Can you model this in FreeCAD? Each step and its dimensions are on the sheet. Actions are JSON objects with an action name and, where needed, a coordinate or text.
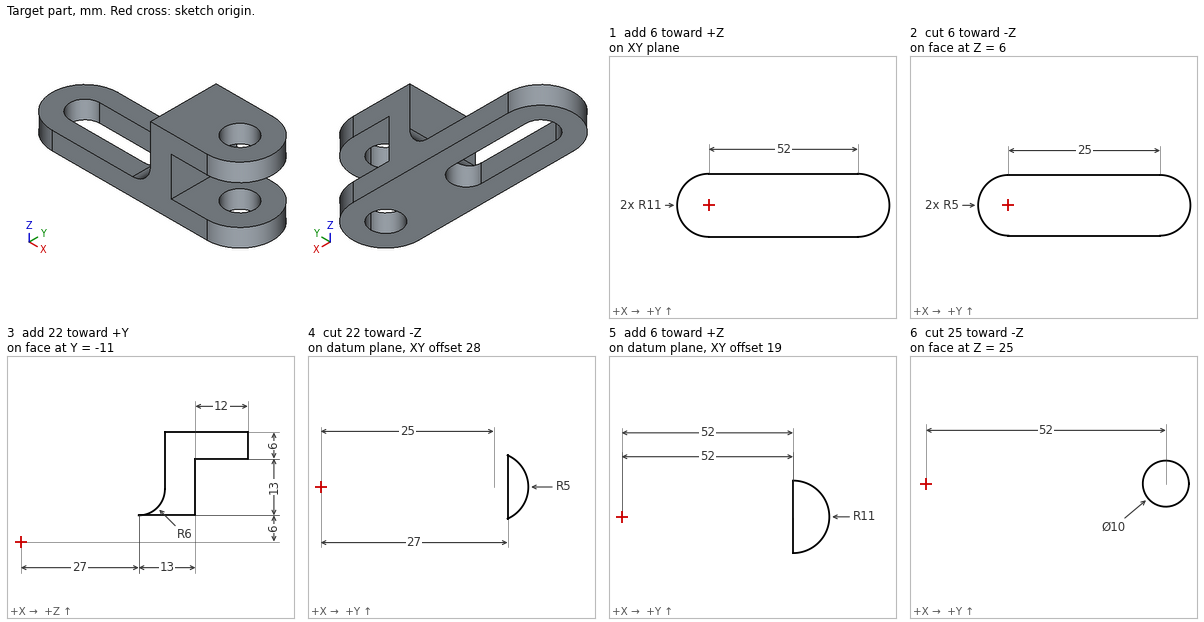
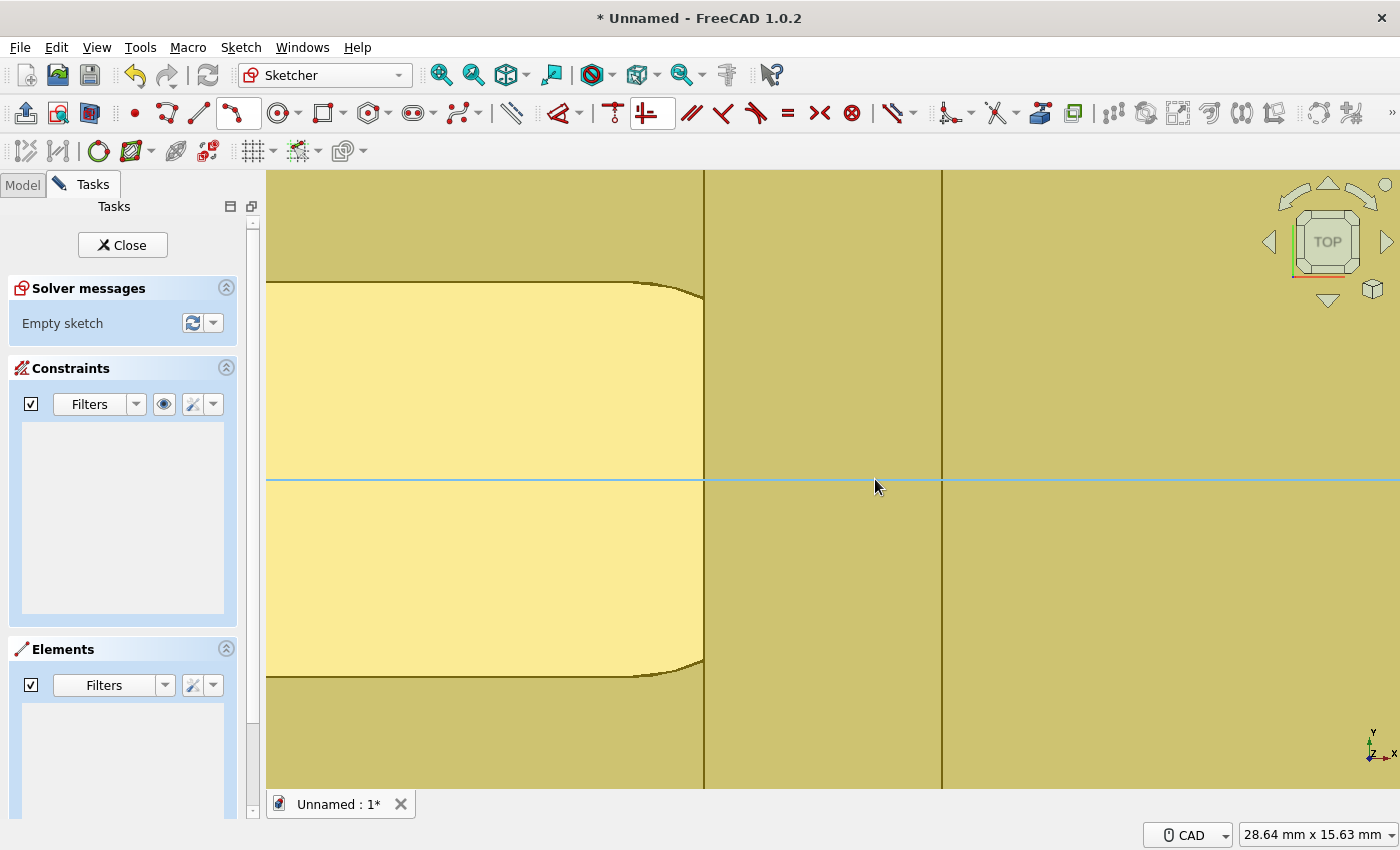
{"action": "left_click", "coordinate": [200, 114]}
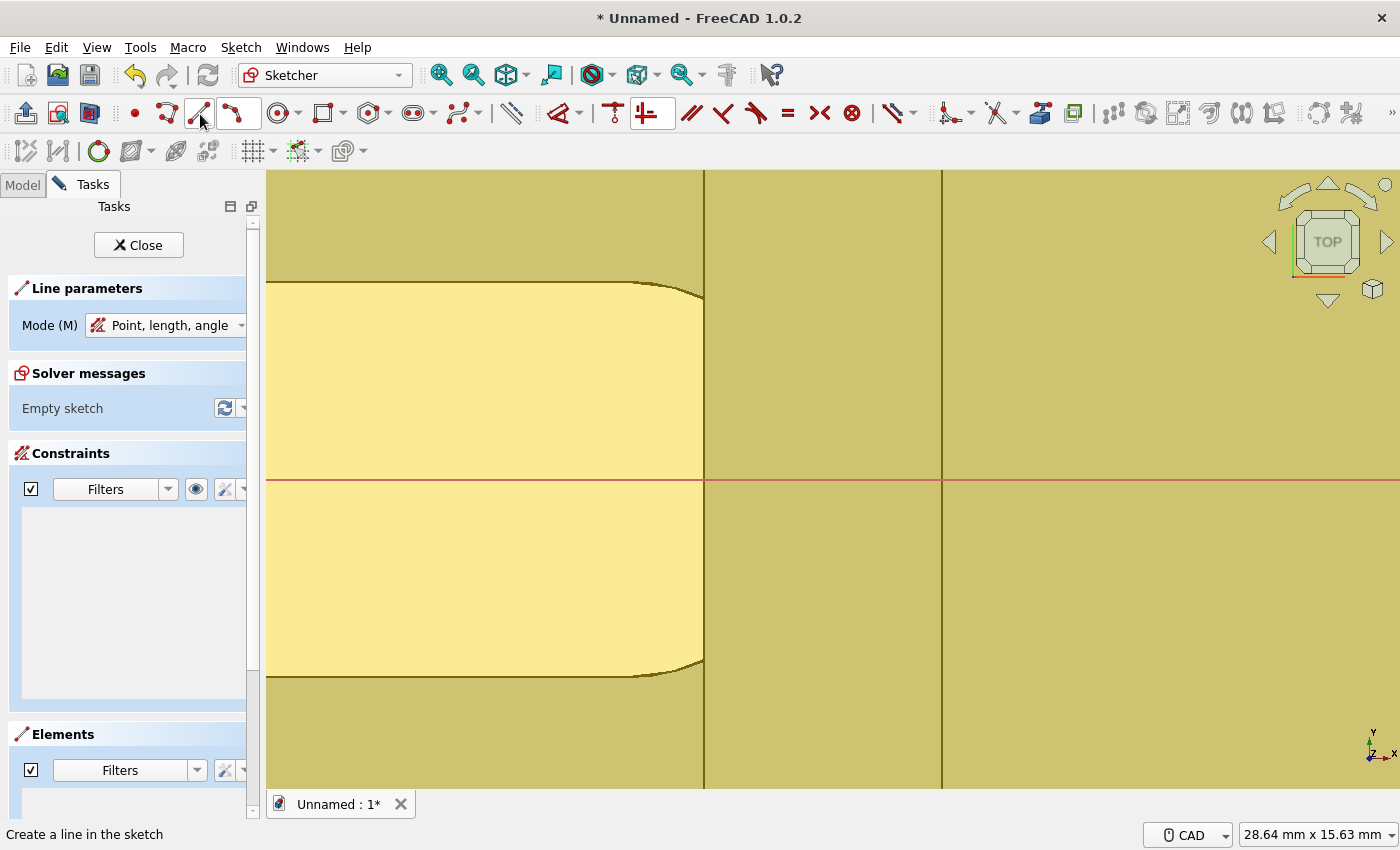
{"action": "left_click", "coordinate": [704, 661]}
{"action": "left_click", "coordinate": [704, 298]}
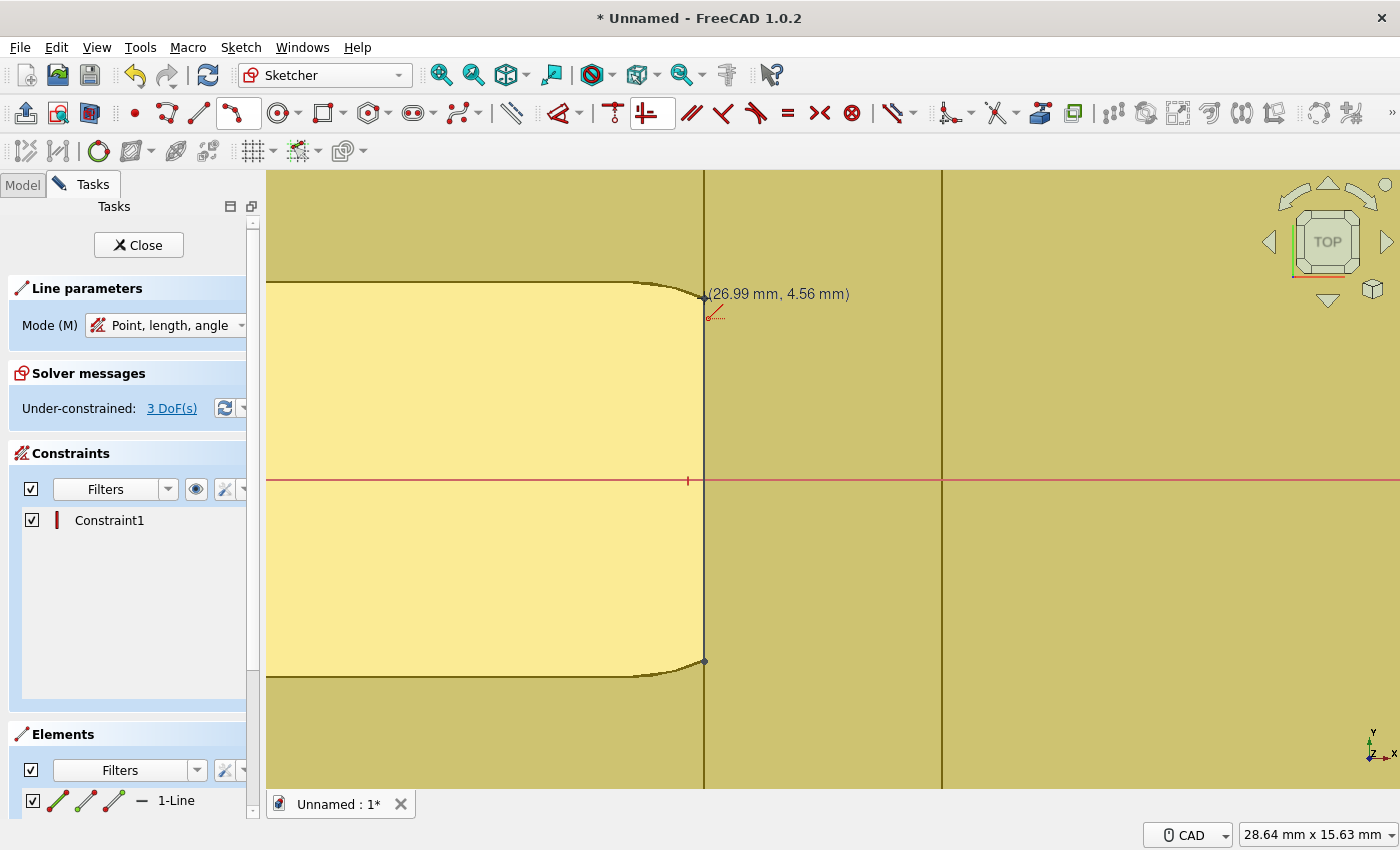
{"action": "left_click", "coordinate": [232, 114]}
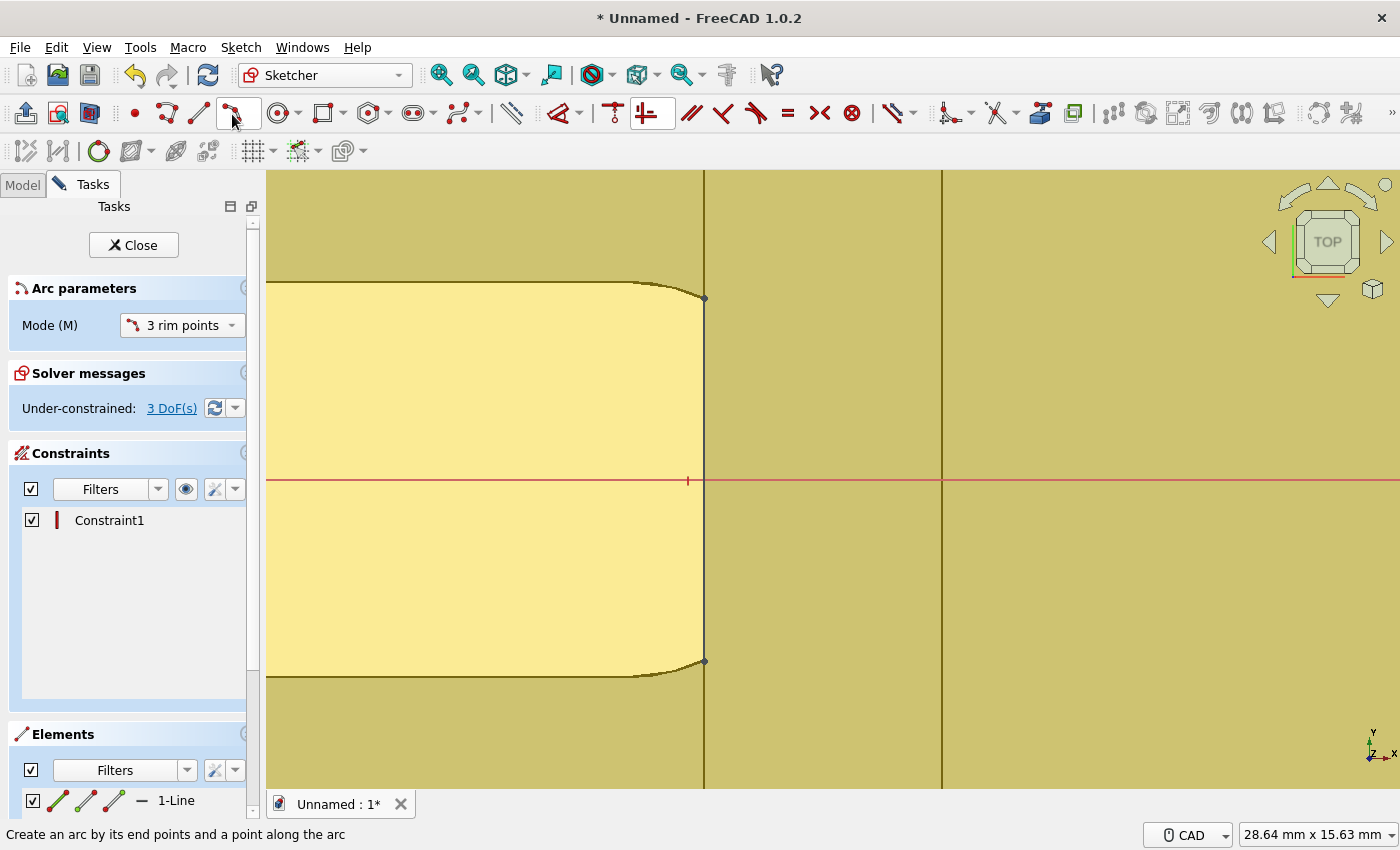
{"action": "left_click", "coordinate": [704, 299]}
{"action": "left_click", "coordinate": [704, 662]}
{"action": "left_click", "coordinate": [818, 525]}
{"action": "key", "text": "Escape"}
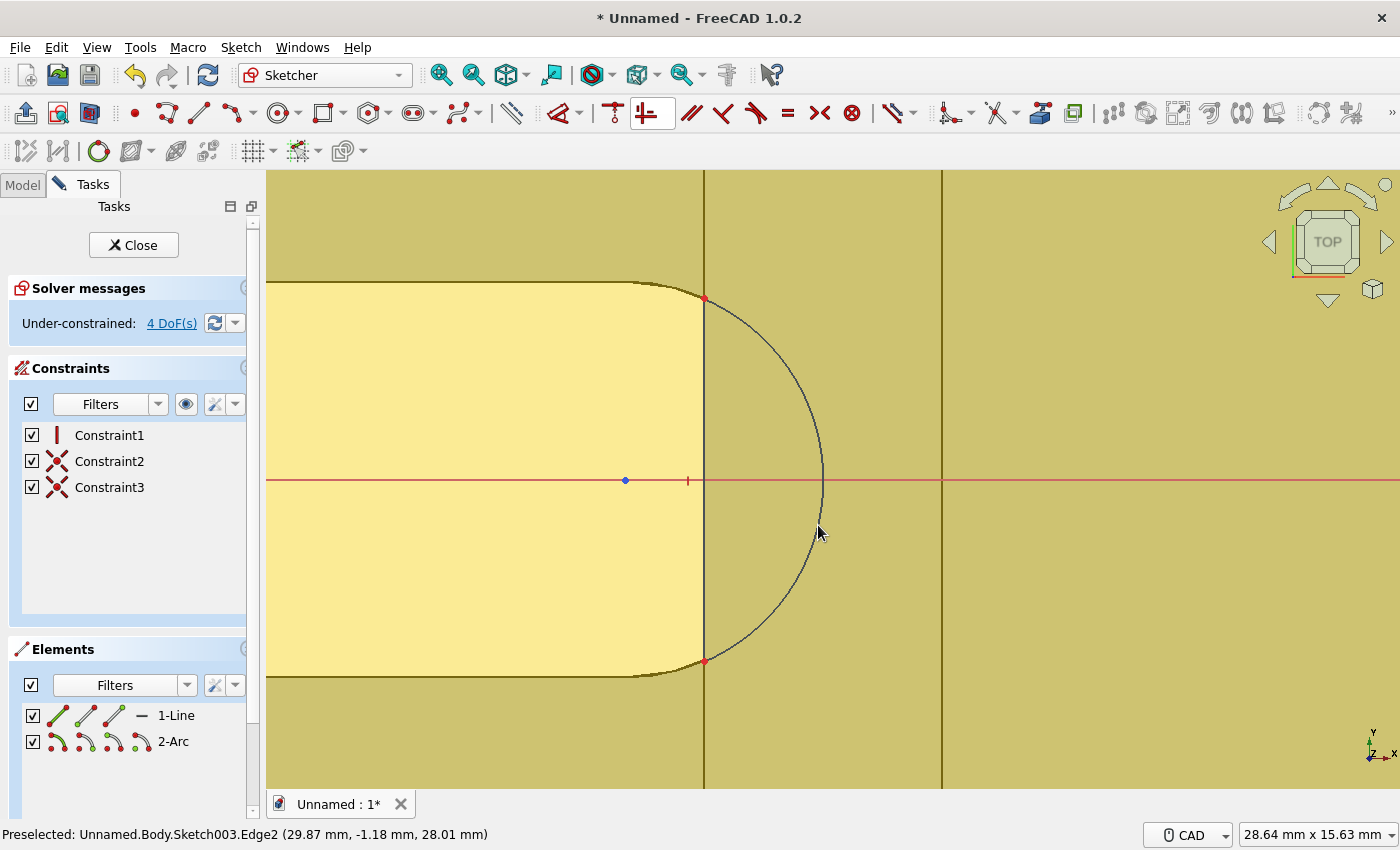
{"action": "left_click", "coordinate": [626, 480]}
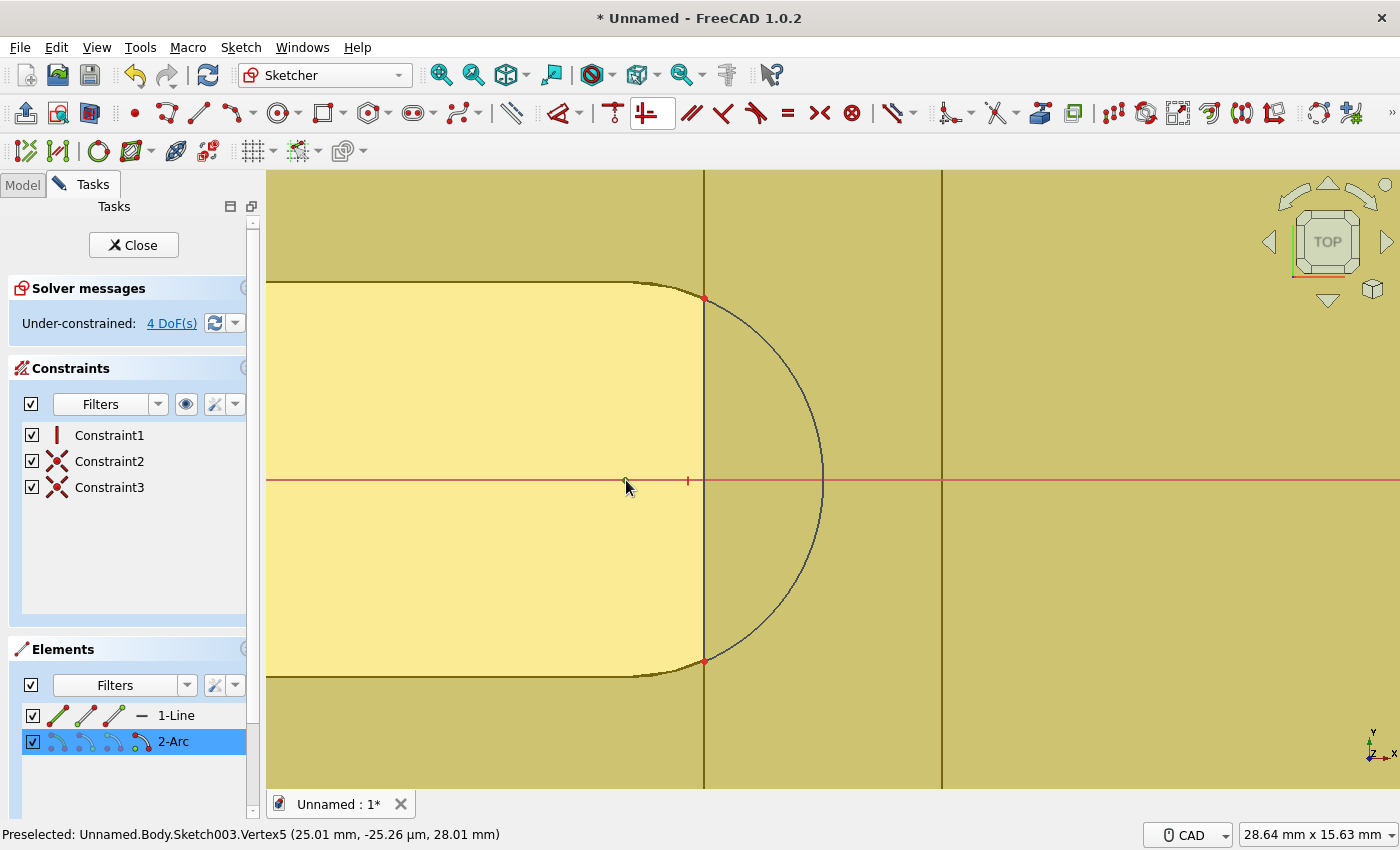
{"action": "left_click", "coordinate": [361, 480]}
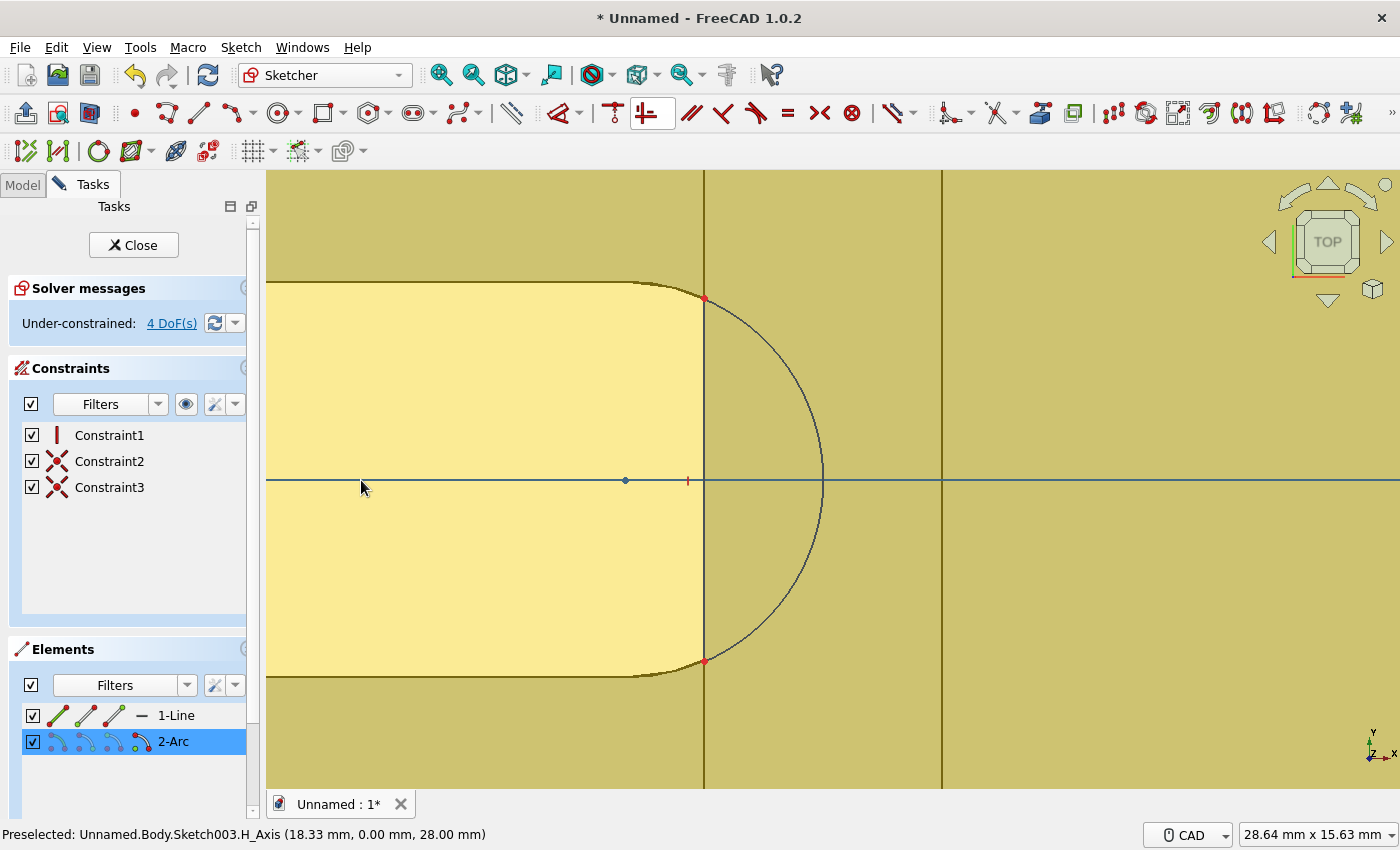
{"action": "left_click", "coordinate": [614, 114]}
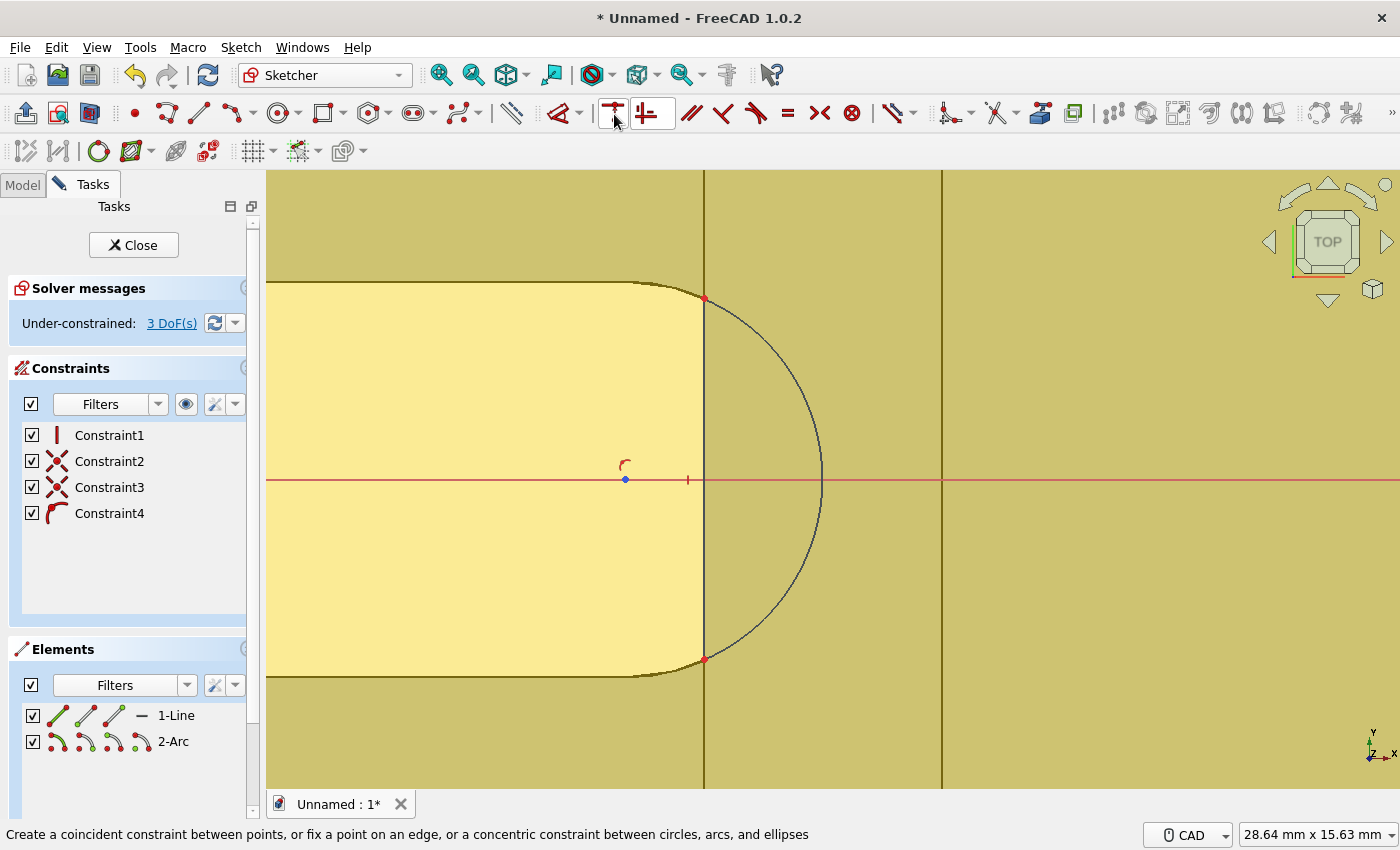
{"action": "left_click", "coordinate": [558, 114]}